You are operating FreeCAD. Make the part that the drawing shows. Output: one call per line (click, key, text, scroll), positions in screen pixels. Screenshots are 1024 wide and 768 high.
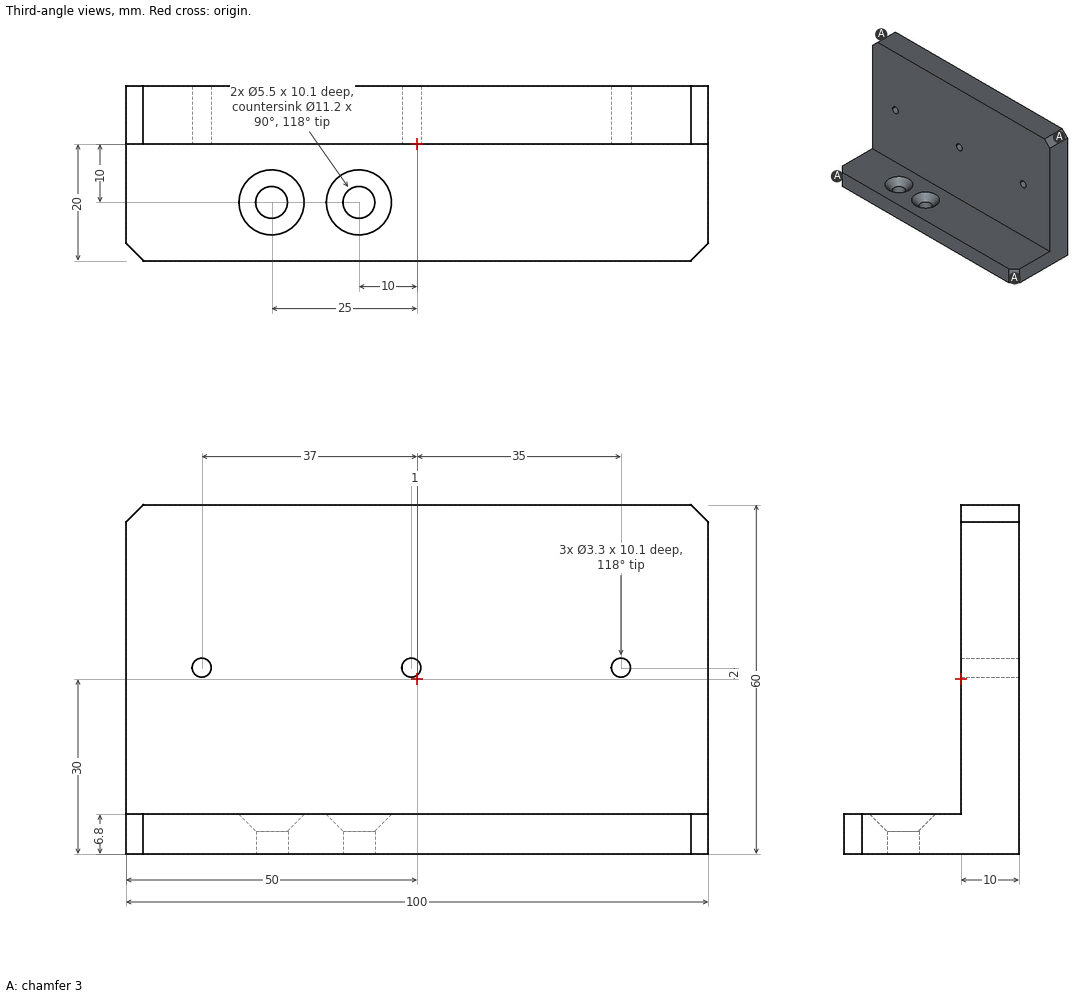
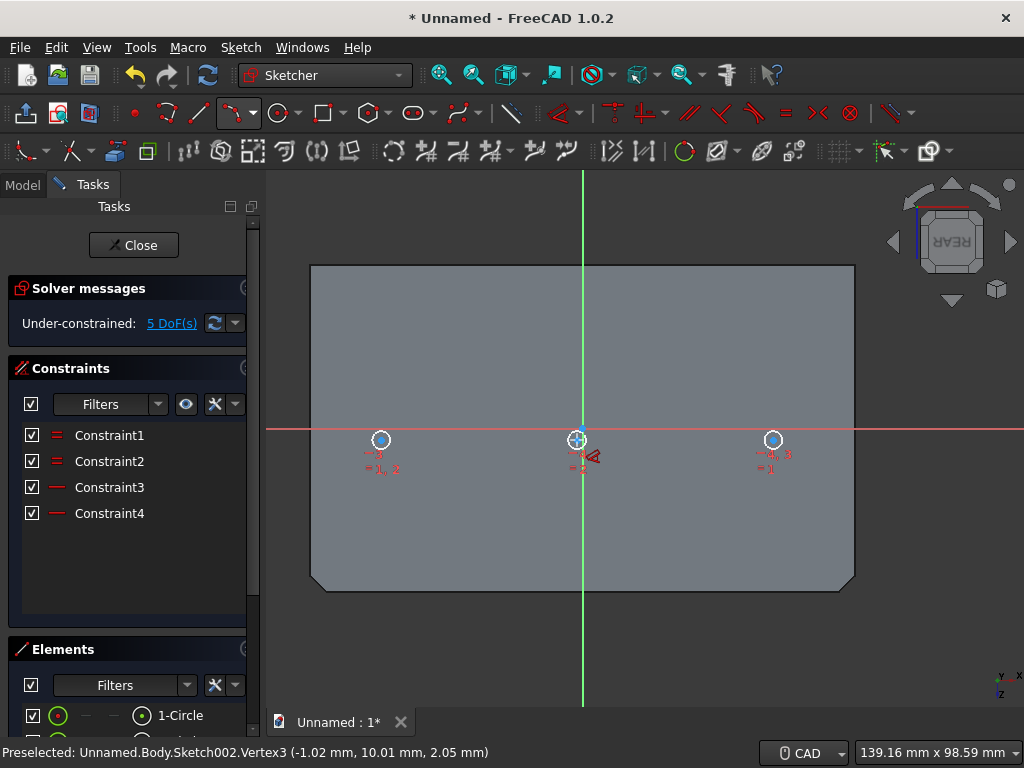
scroll(780, 446, up, 4)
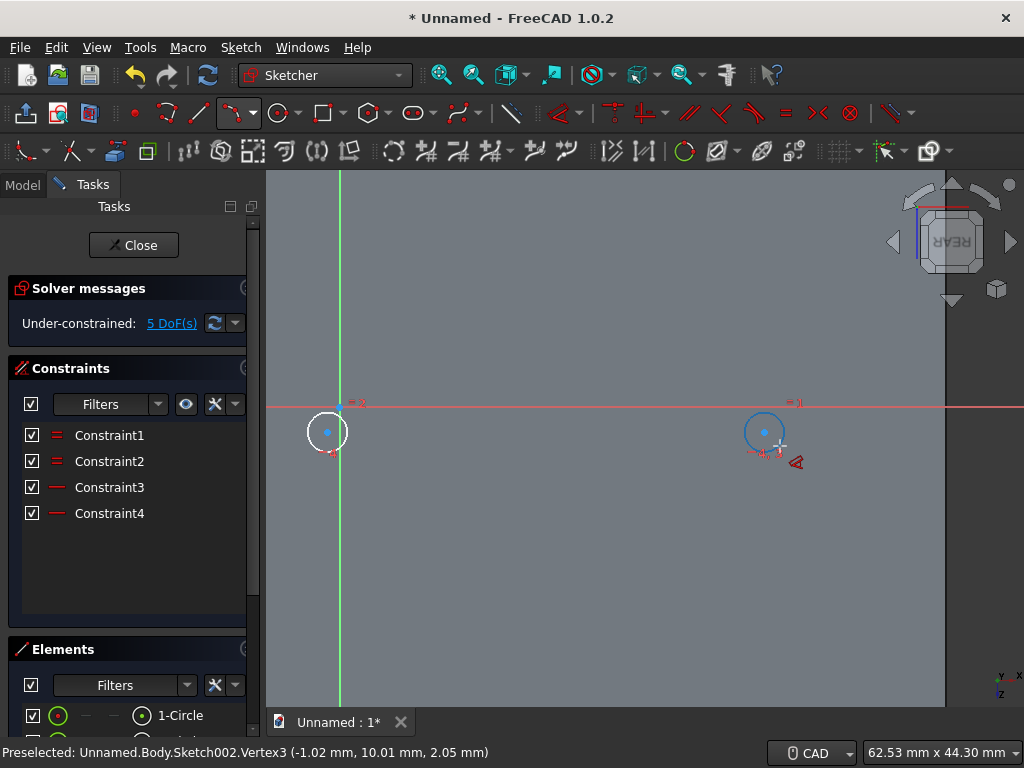
click(778, 446)
click(800, 469)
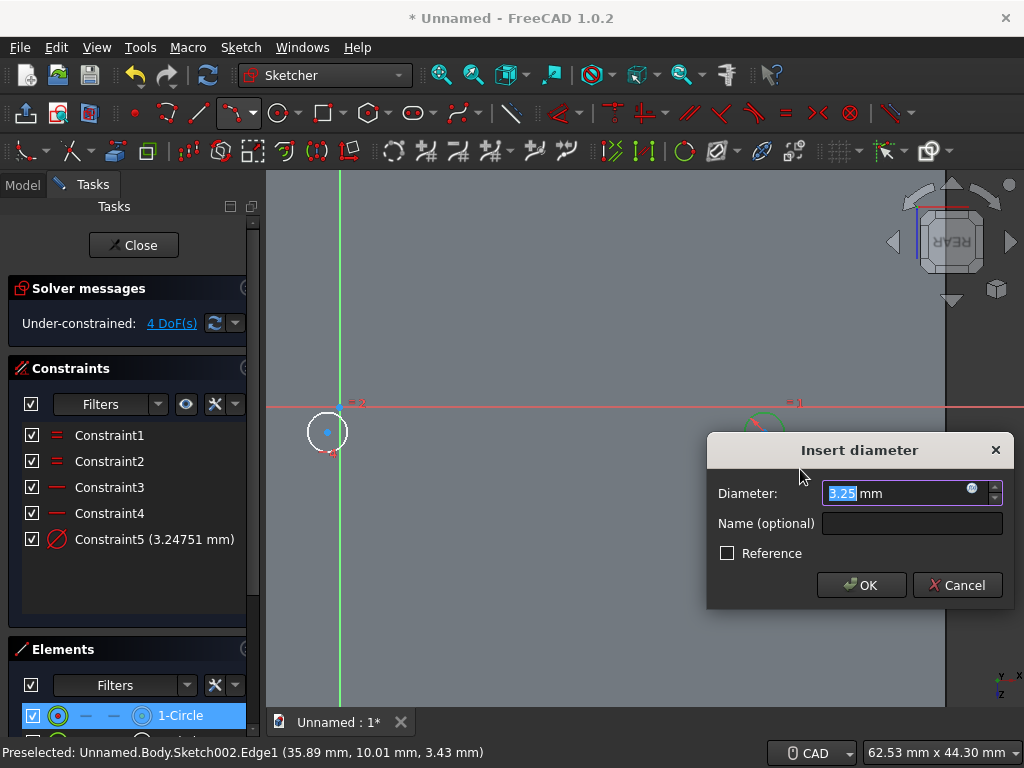
text(3.3)
key(Return)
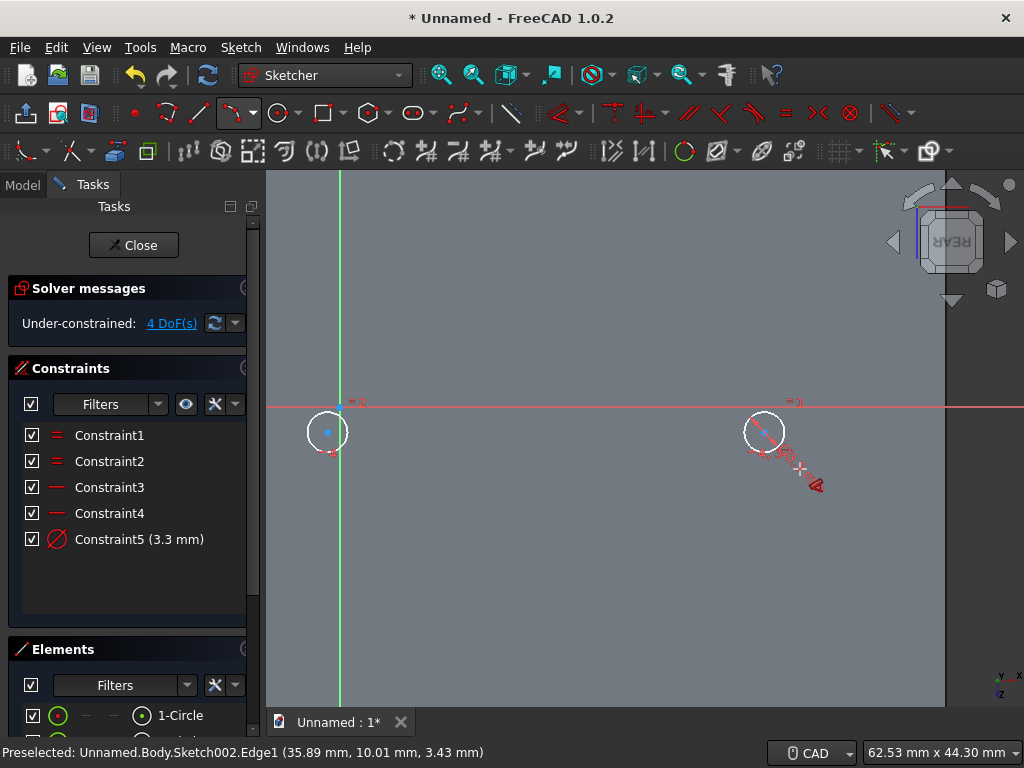
scroll(764, 432, up, 3)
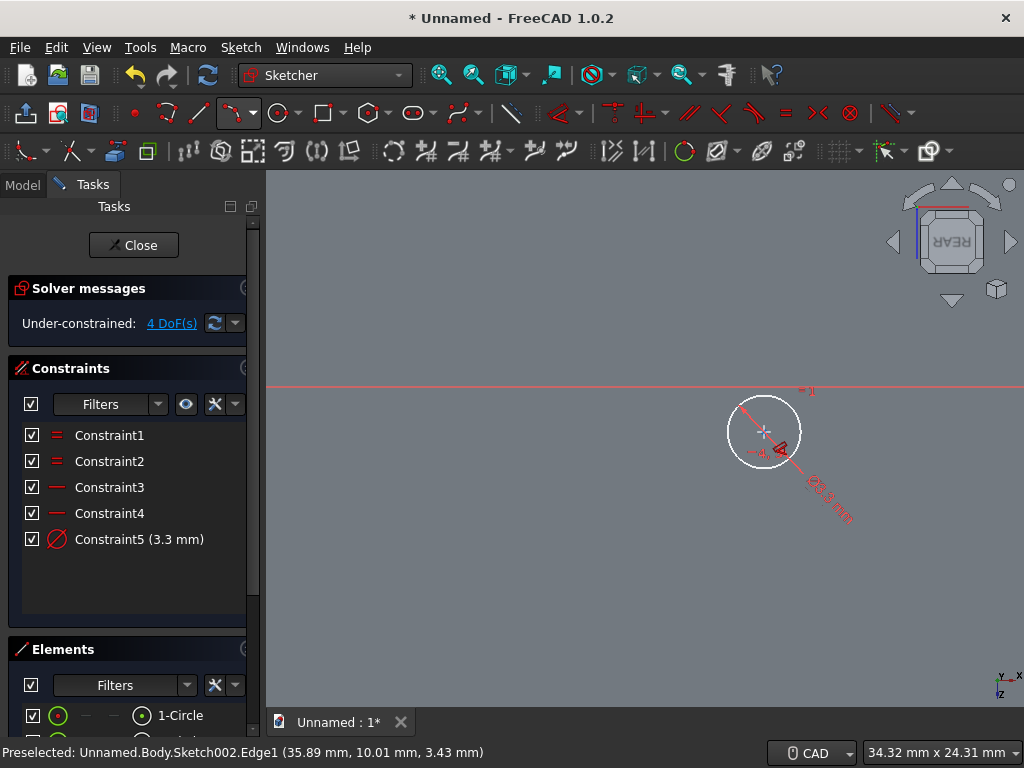
click(764, 432)
click(822, 409)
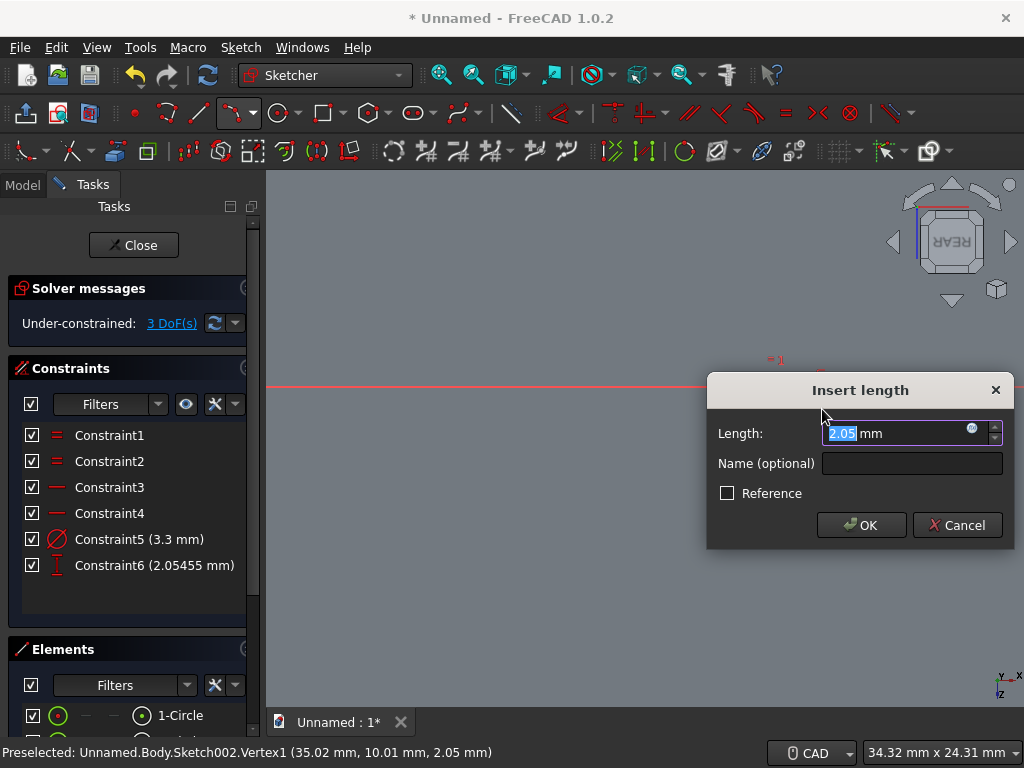
text(2)
key(Return)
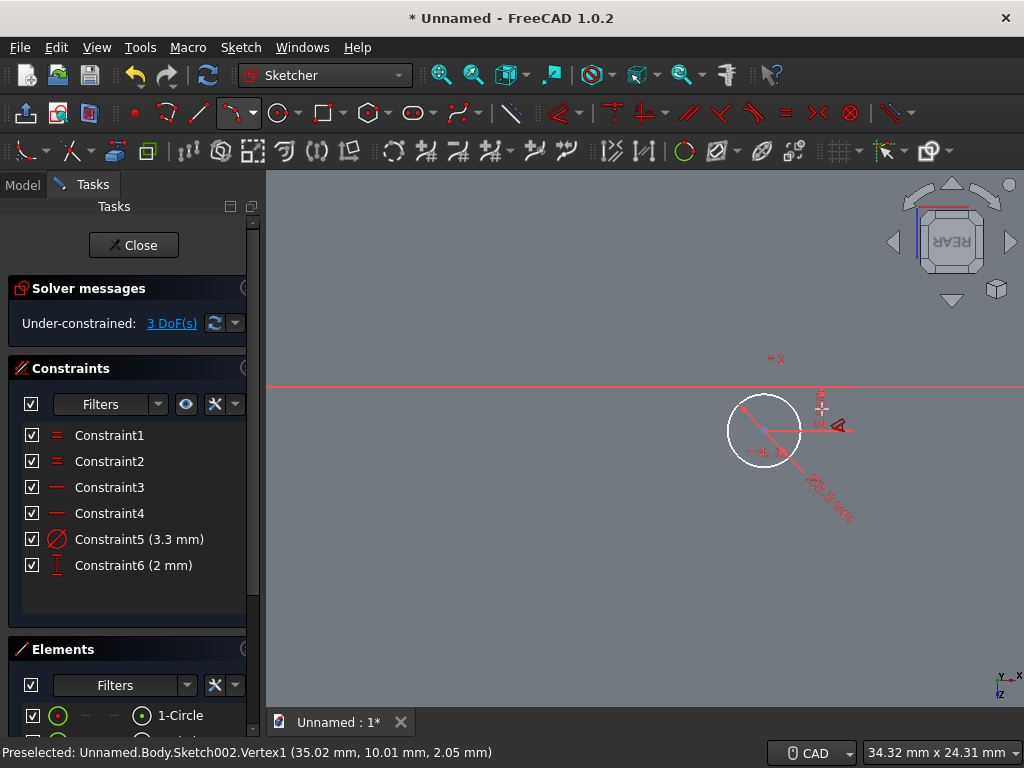
scroll(776, 442, down, 7)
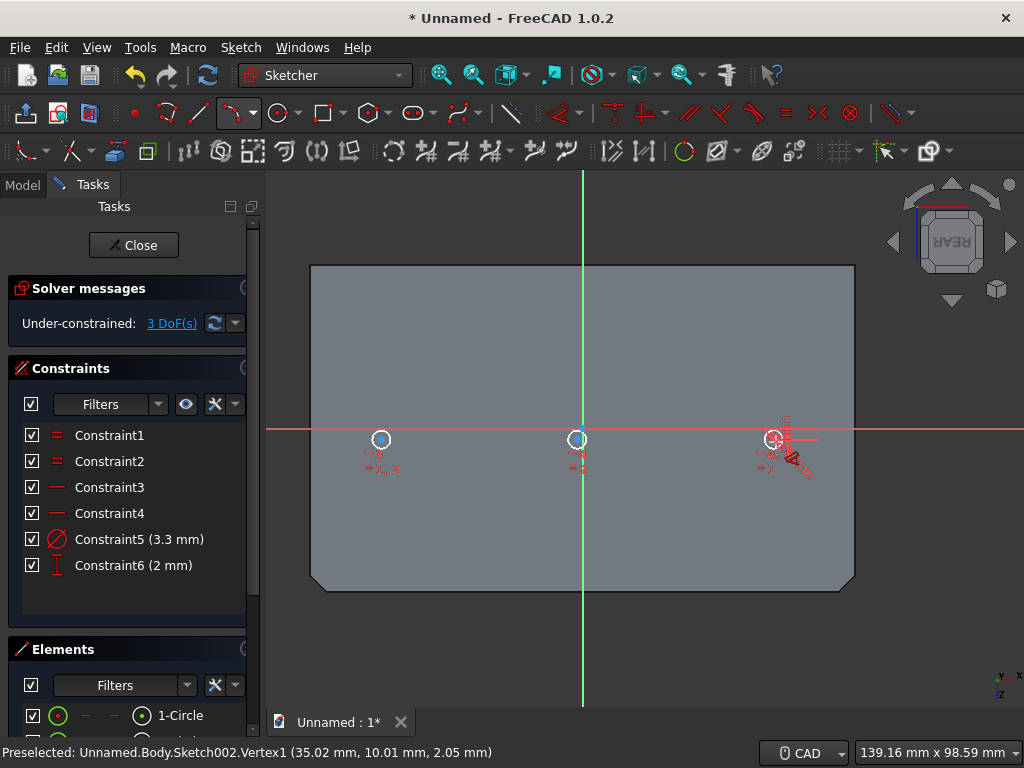
scroll(577, 440, up, 10)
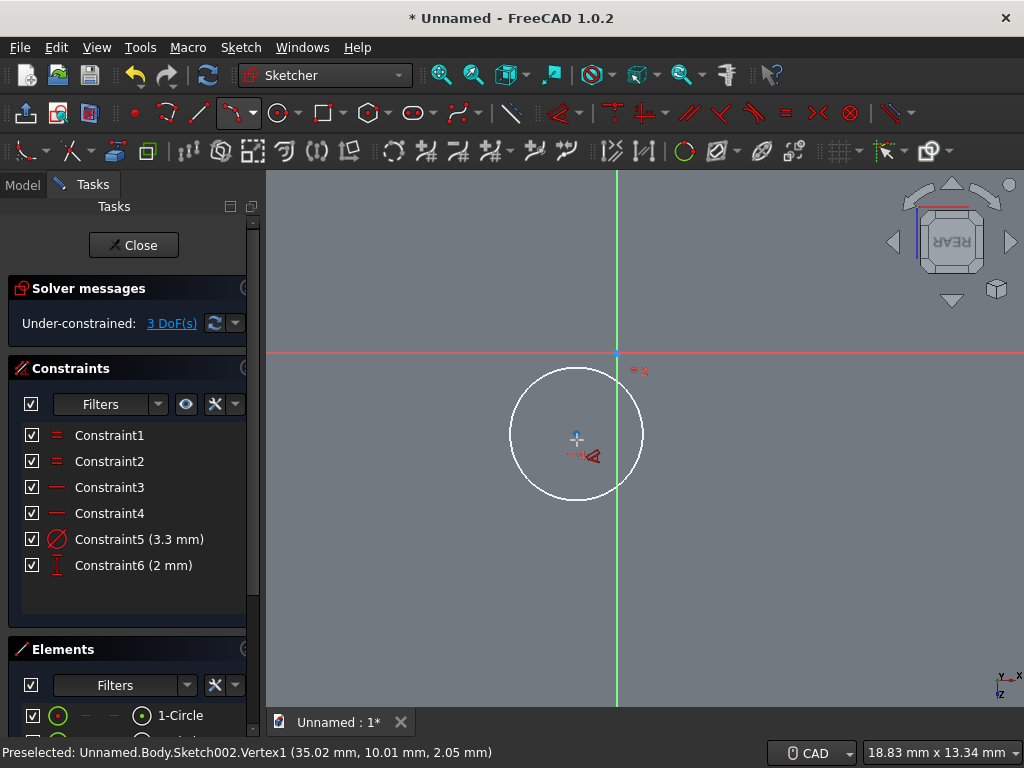
click(576, 434)
click(597, 319)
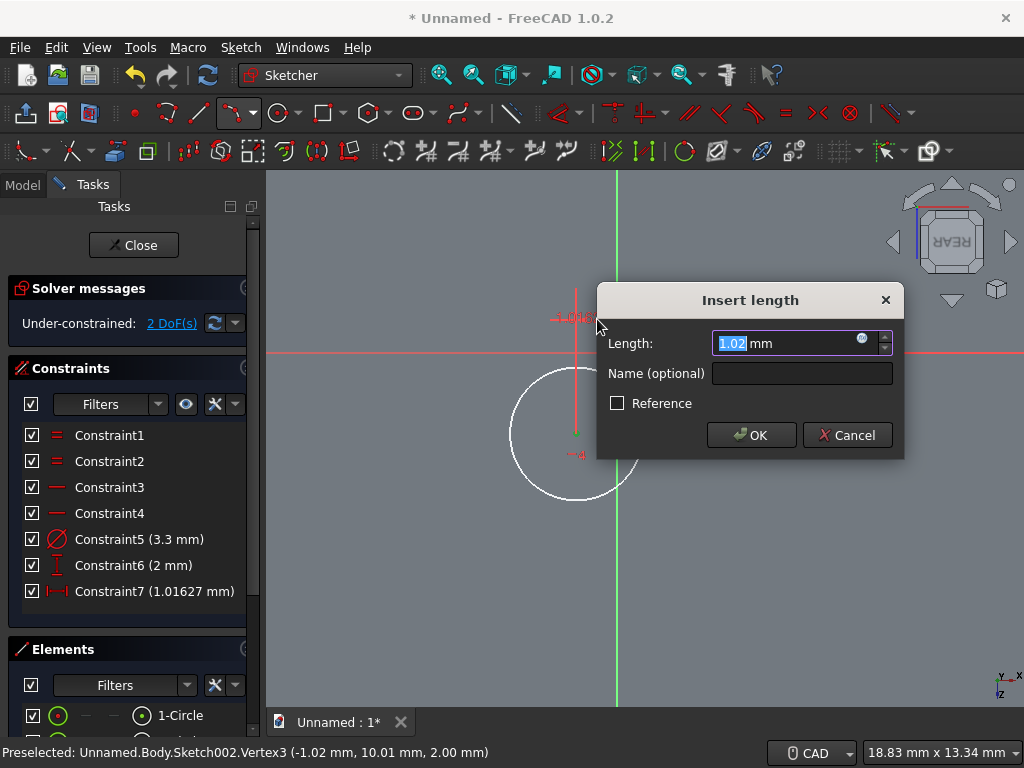
text(1)
key(Return)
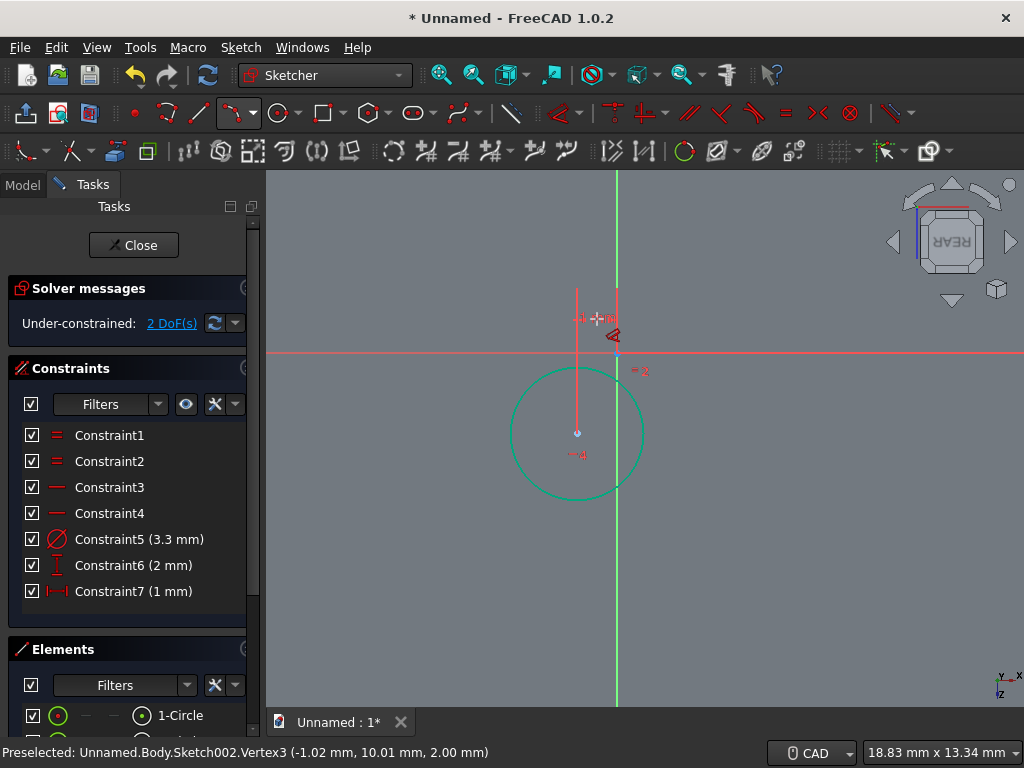
scroll(576, 440, down, 10)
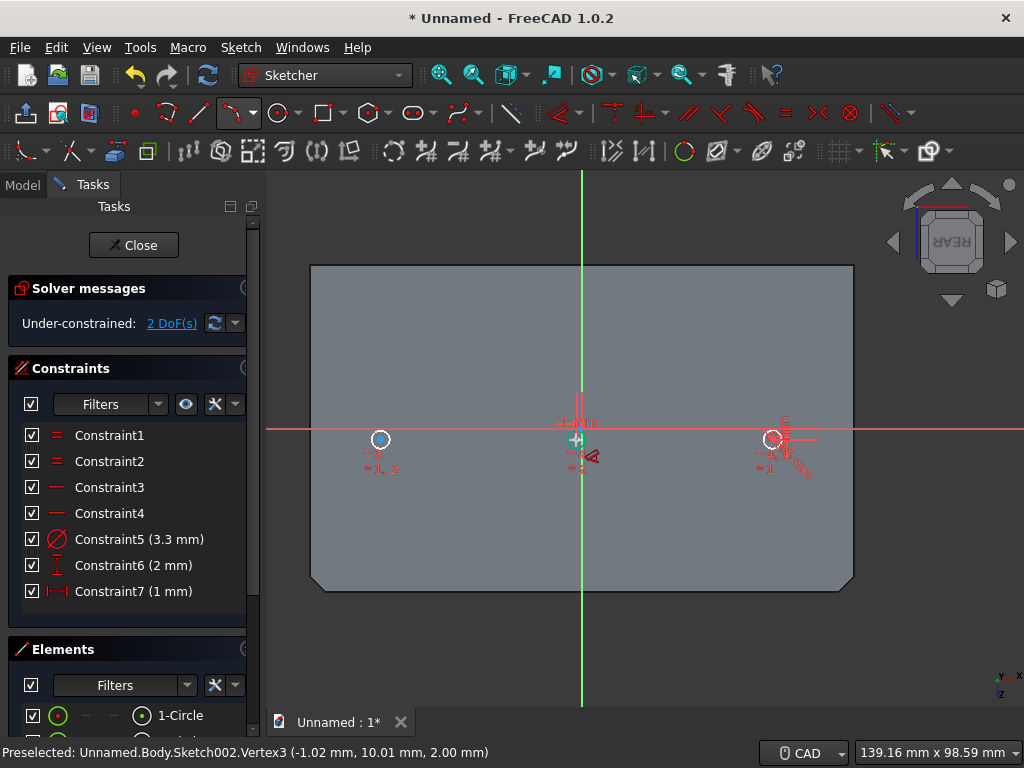
click(773, 440)
click(677, 395)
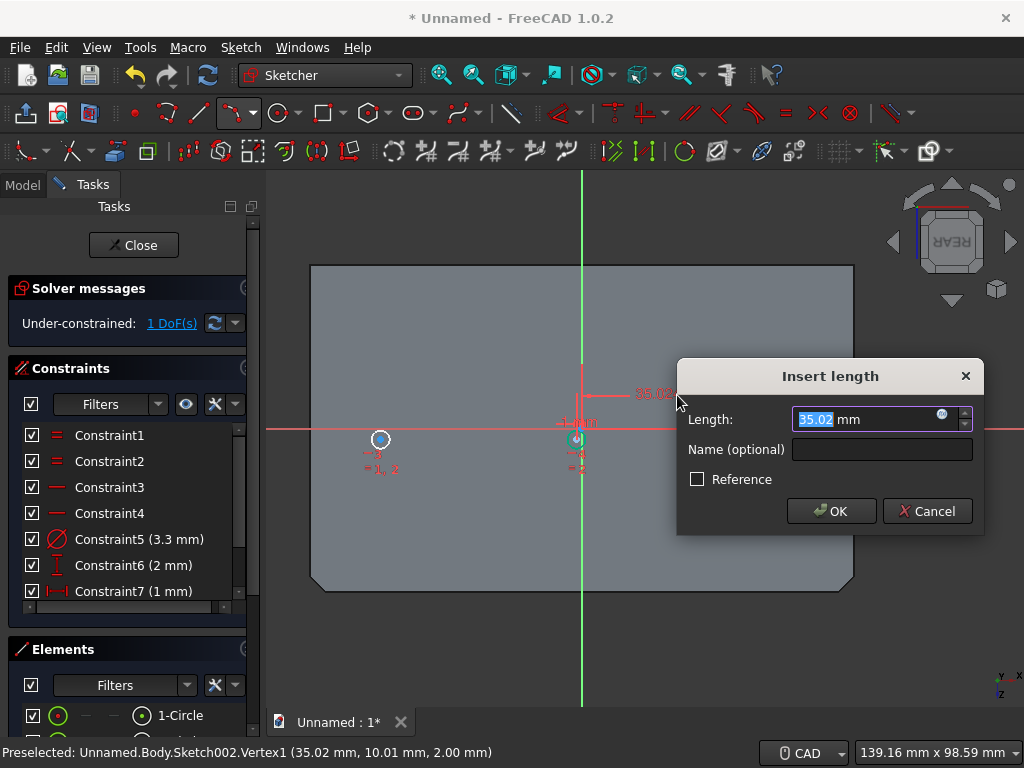
text(35)
key(Return)